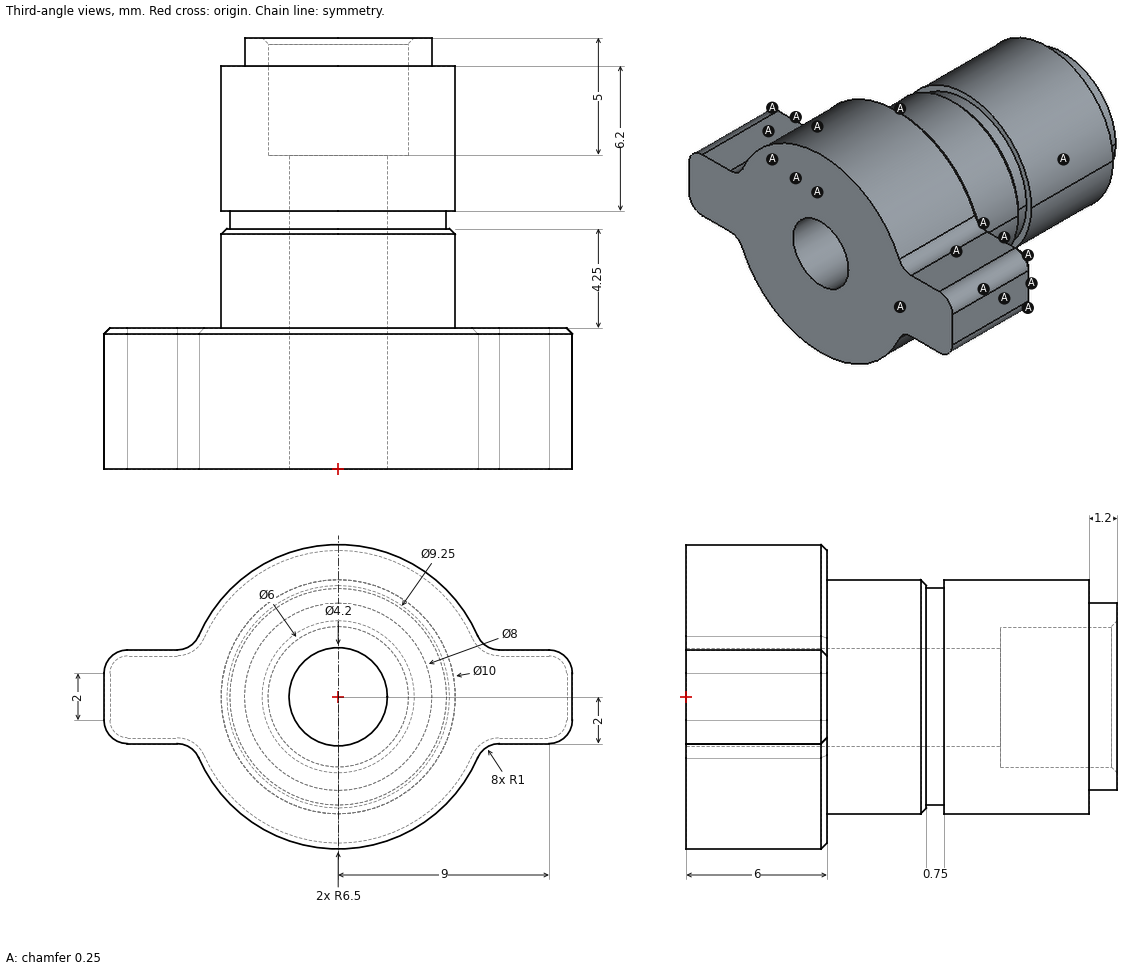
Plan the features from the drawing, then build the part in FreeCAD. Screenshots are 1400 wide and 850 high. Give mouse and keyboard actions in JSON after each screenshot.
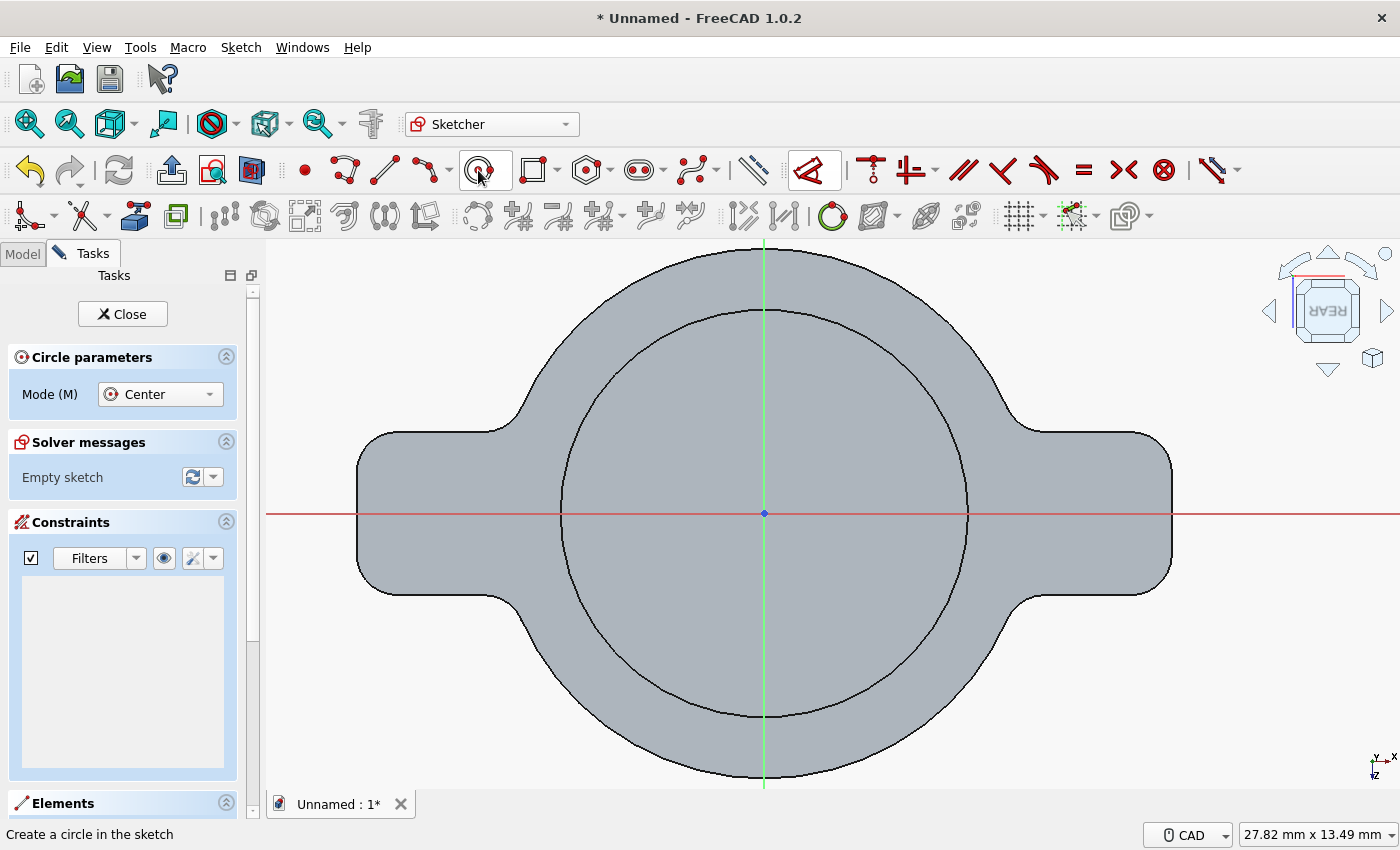
{"action": "left_click", "coordinate": [764, 514]}
{"action": "mouse_move", "coordinate": [898, 380]}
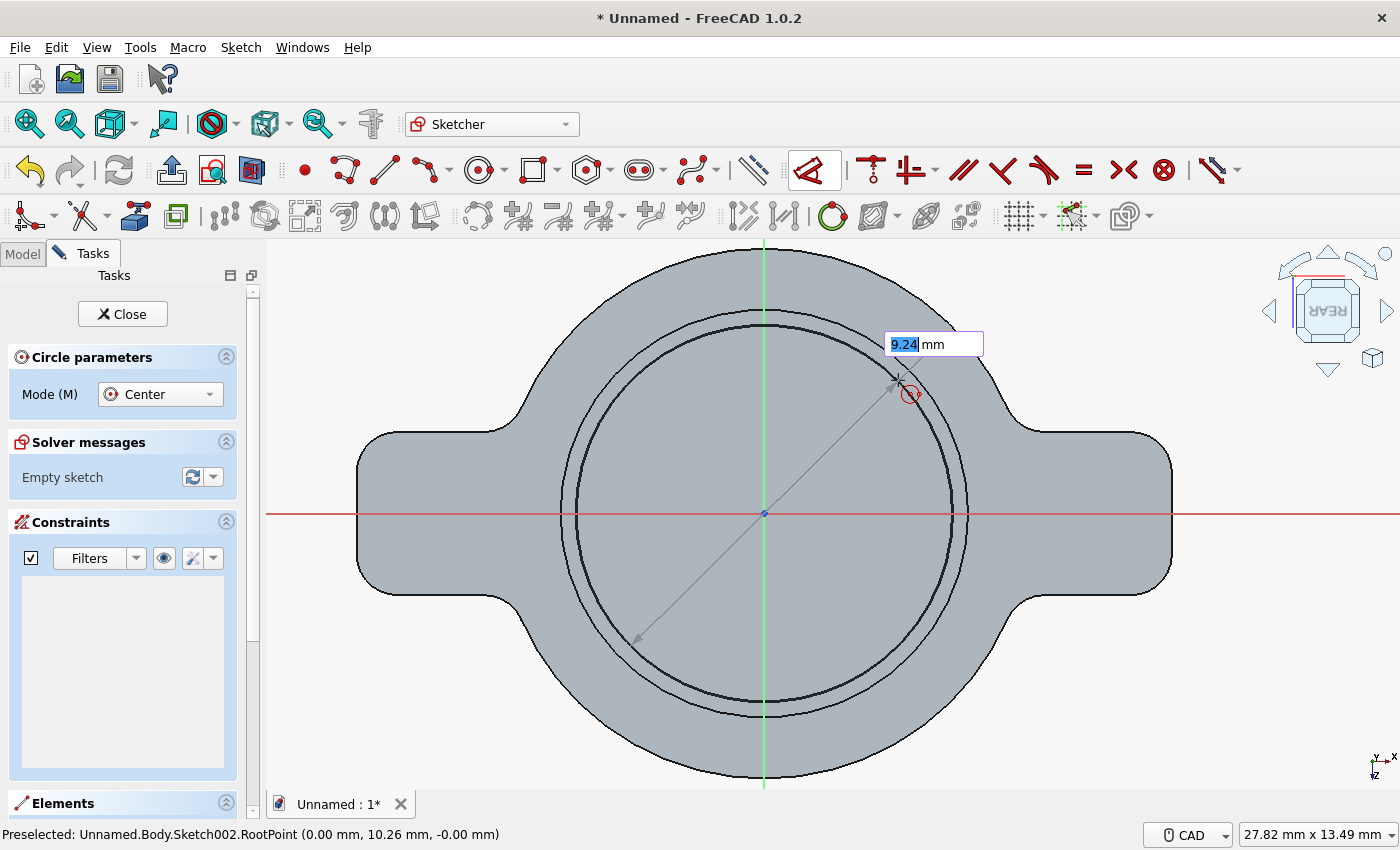
{"action": "type", "text": "9.25"}
{"action": "key", "text": "Return"}
{"action": "key", "text": "Escape"}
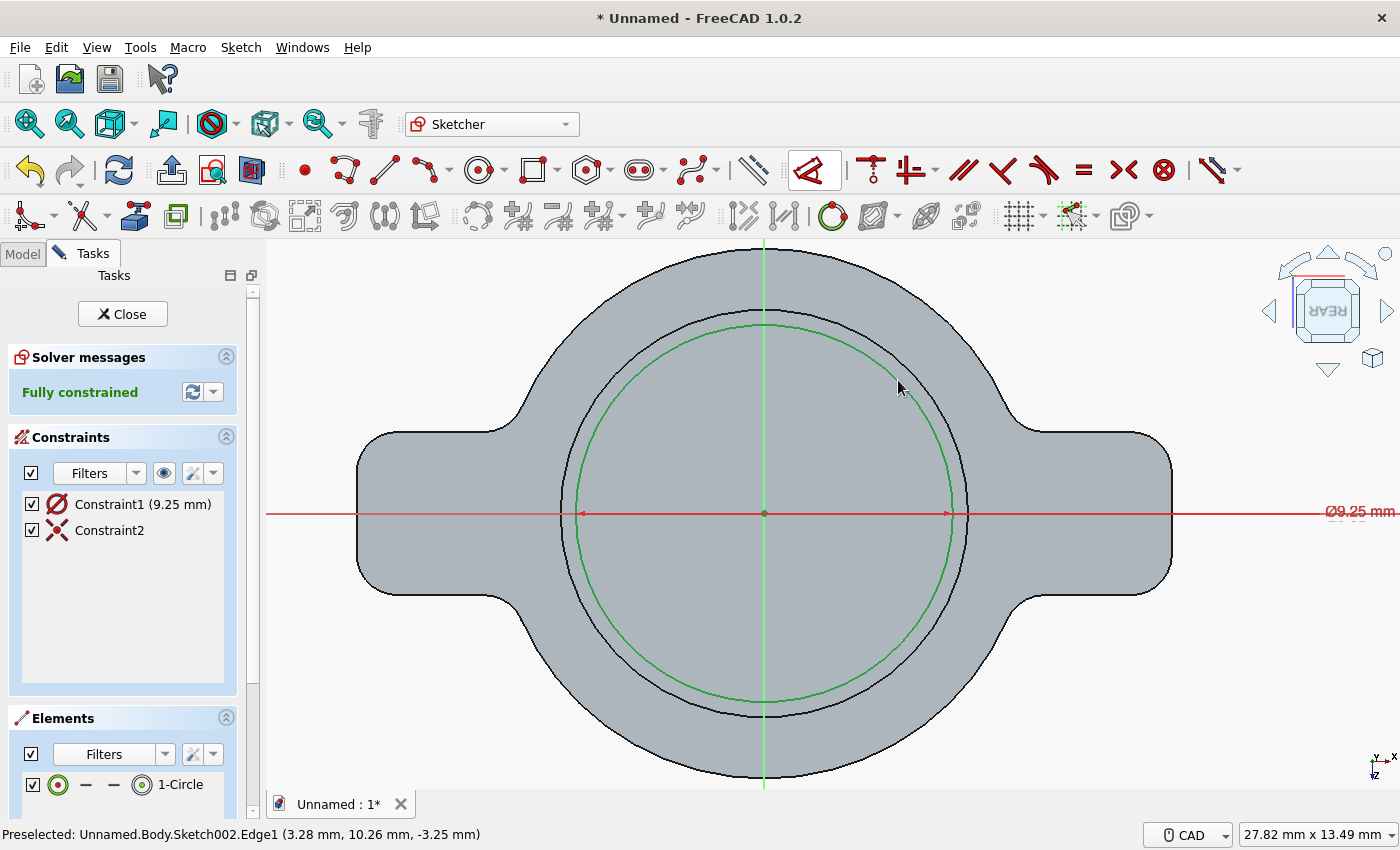
{"action": "left_click", "coordinate": [123, 314]}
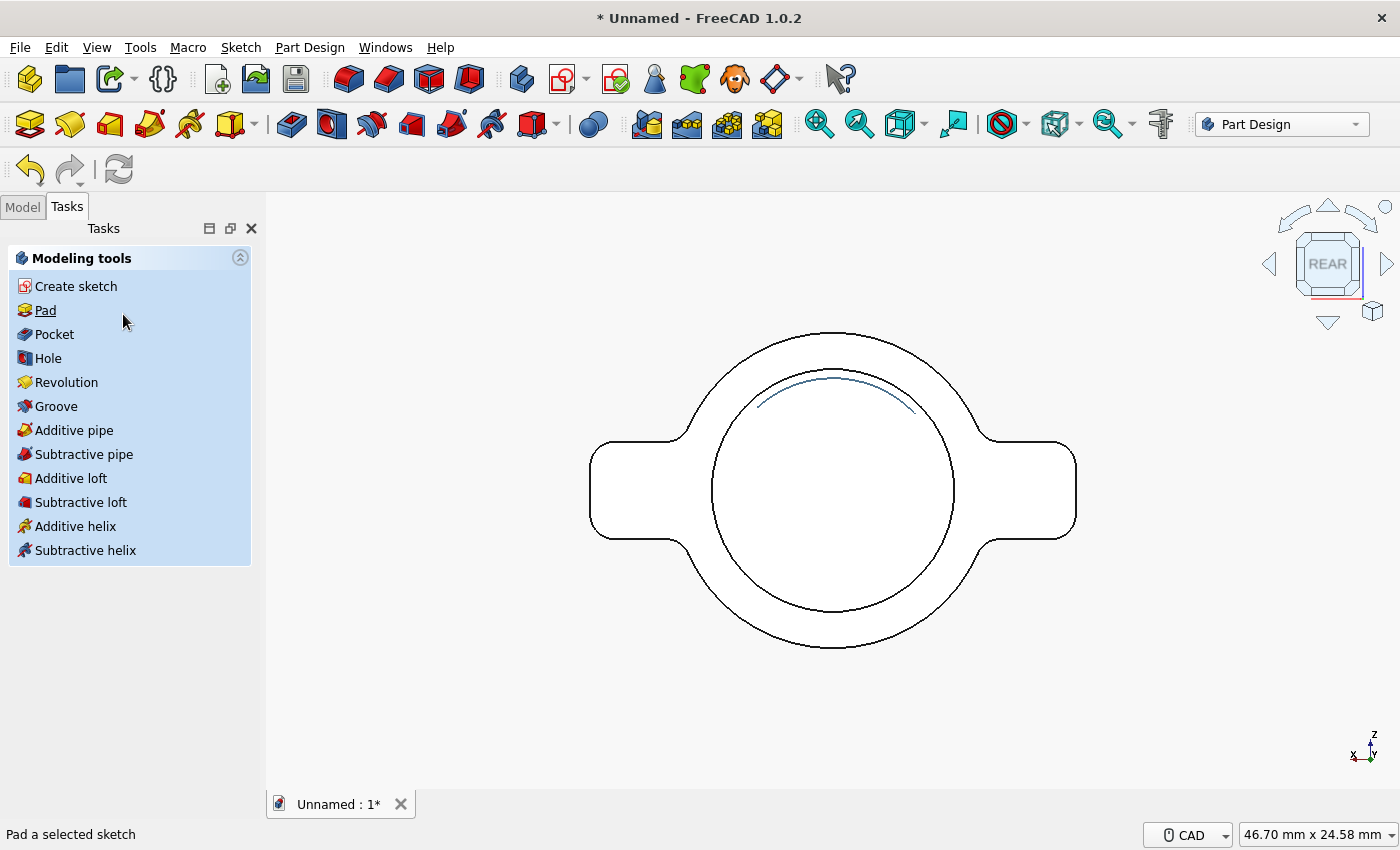
{"action": "left_click", "coordinate": [30, 124]}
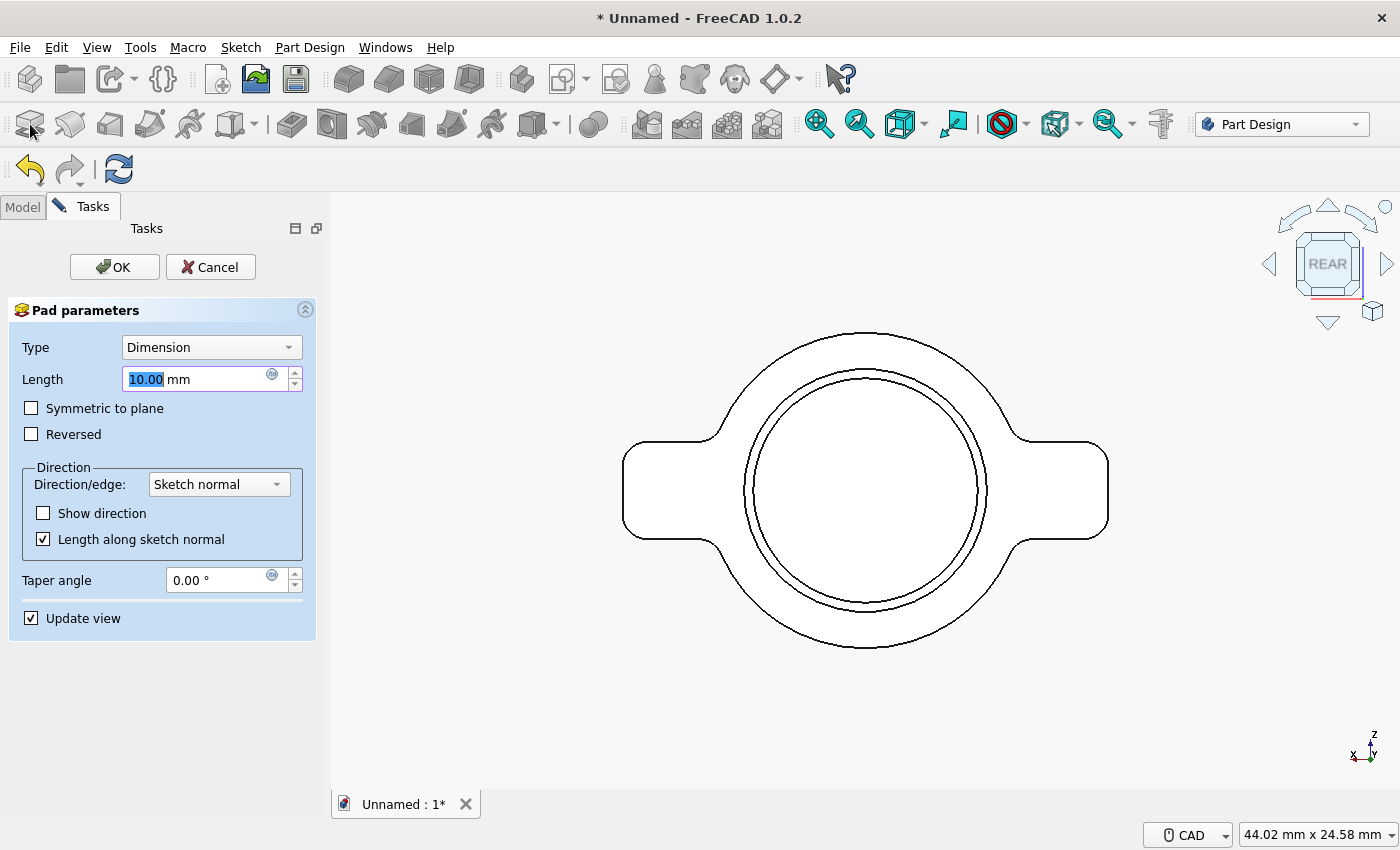
{"action": "type", "text": "0.75"}
{"action": "key", "text": "Tab"}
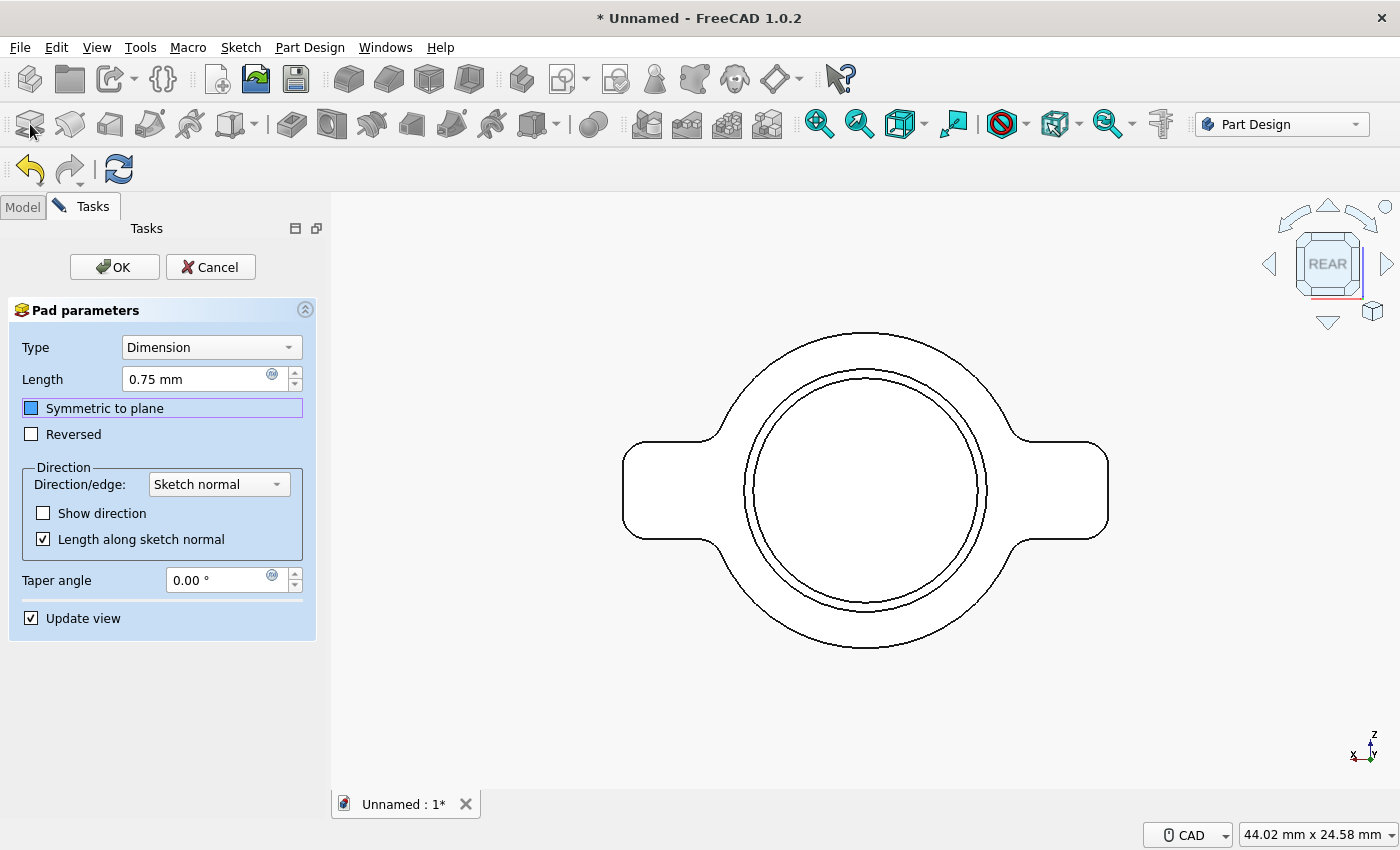
{"action": "left_click", "coordinate": [115, 267]}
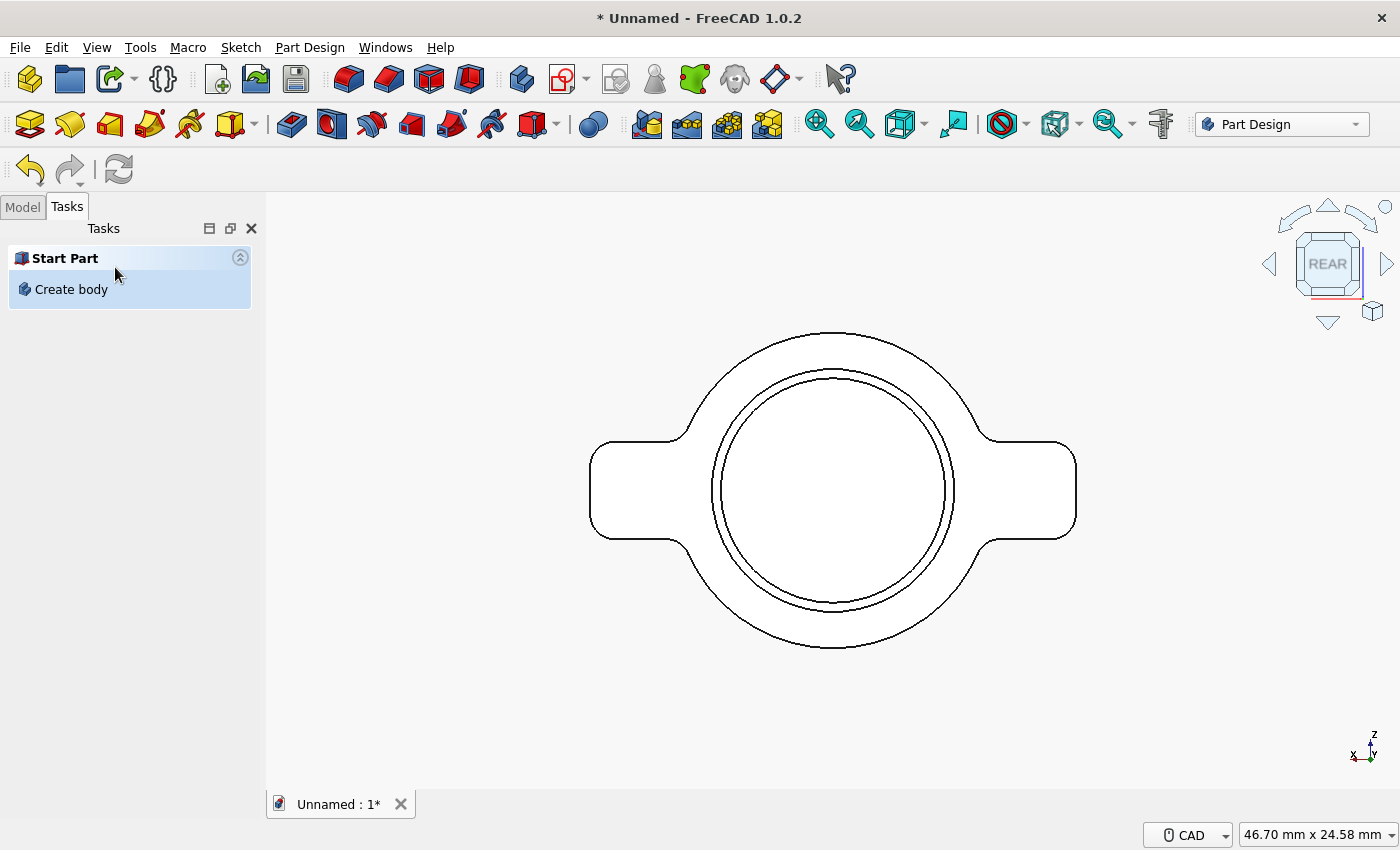
{"action": "left_click", "coordinate": [833, 490]}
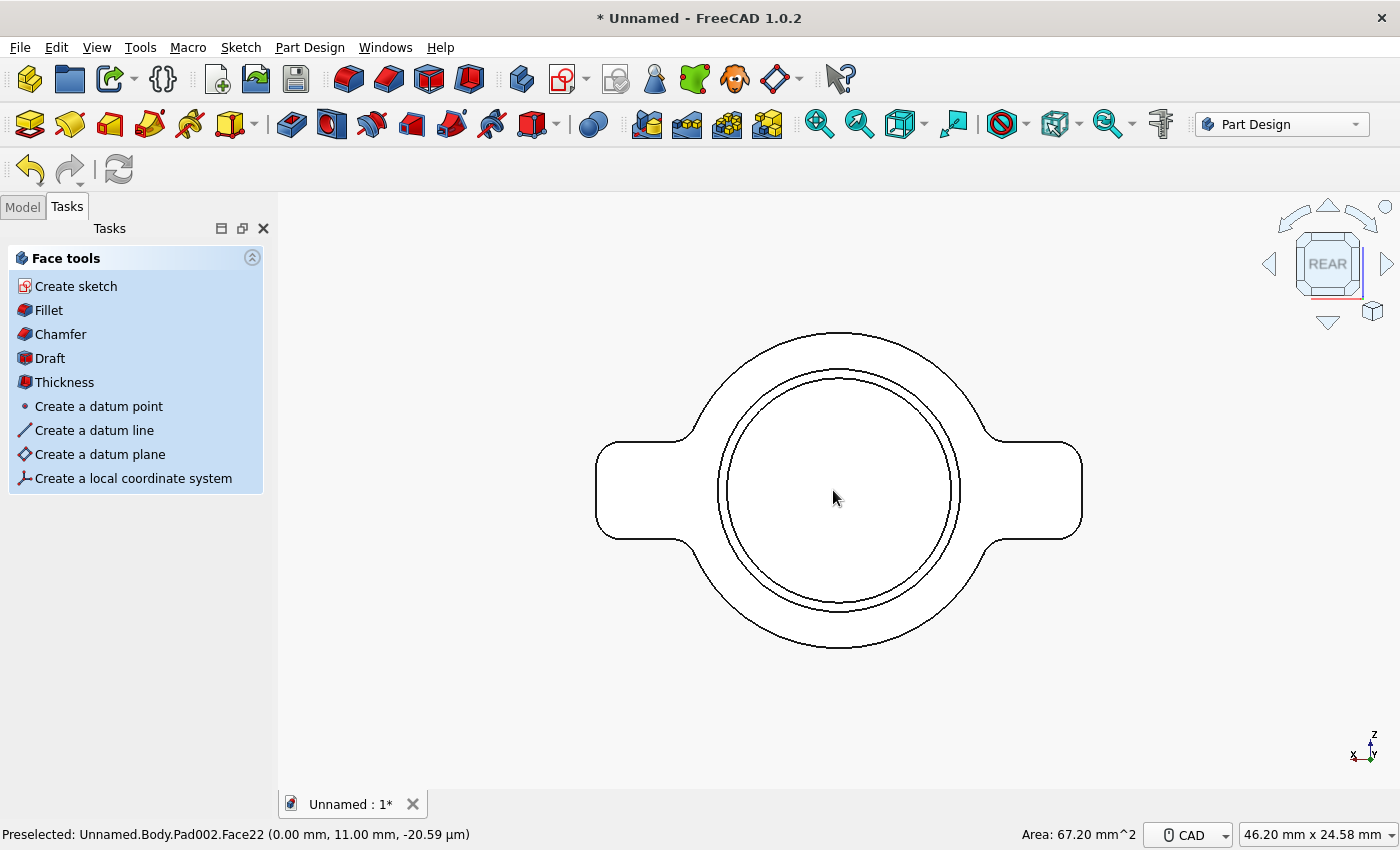
{"action": "left_click", "coordinate": [562, 80]}